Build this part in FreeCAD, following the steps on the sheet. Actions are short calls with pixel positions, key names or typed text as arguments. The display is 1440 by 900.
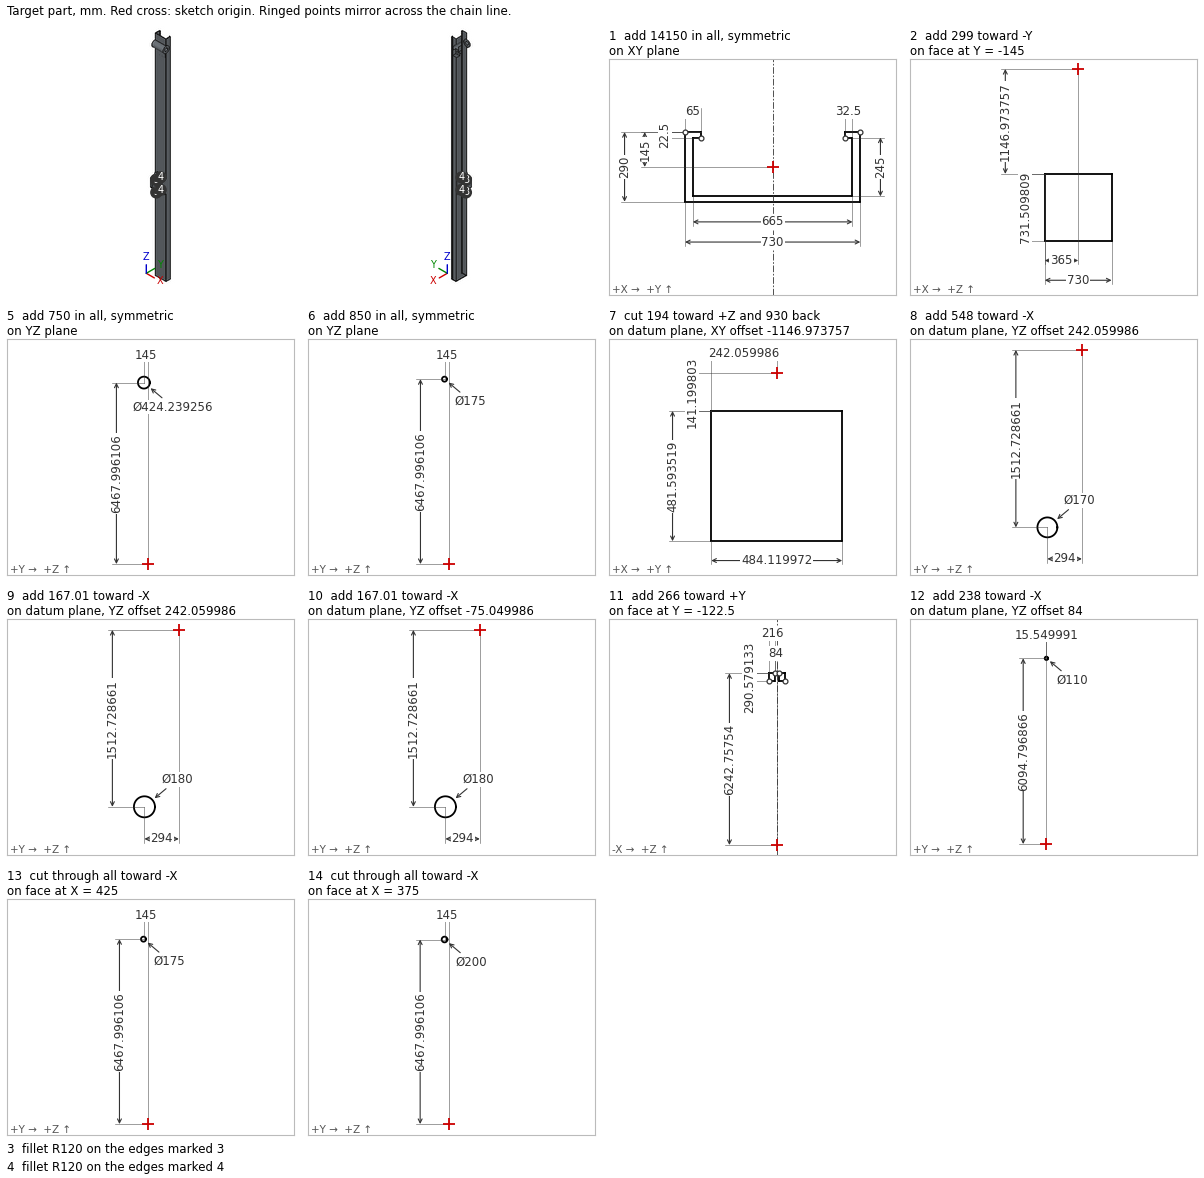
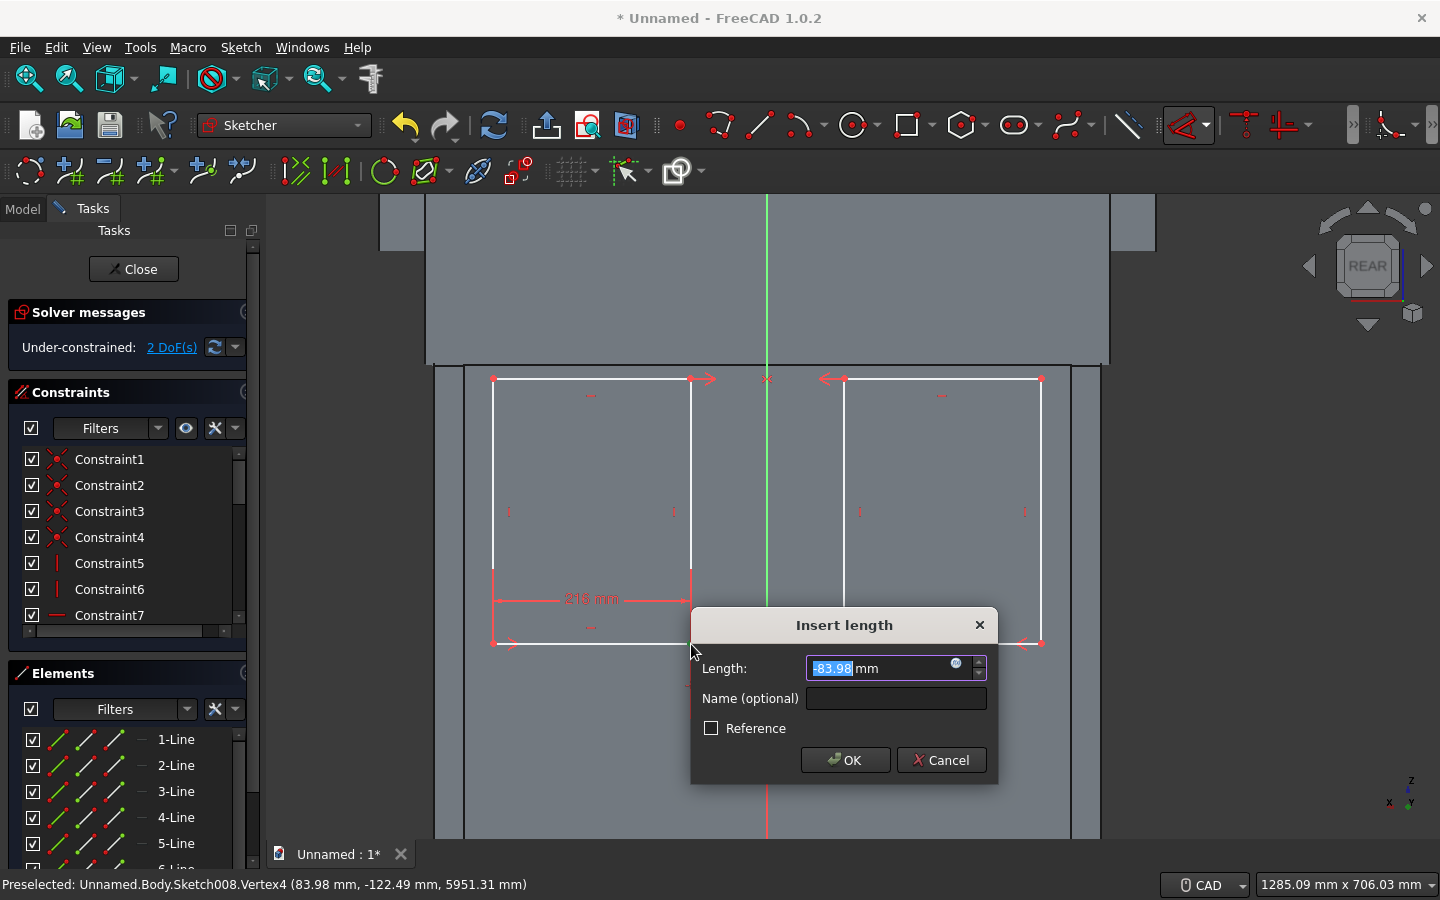
text(-84)
key(Return)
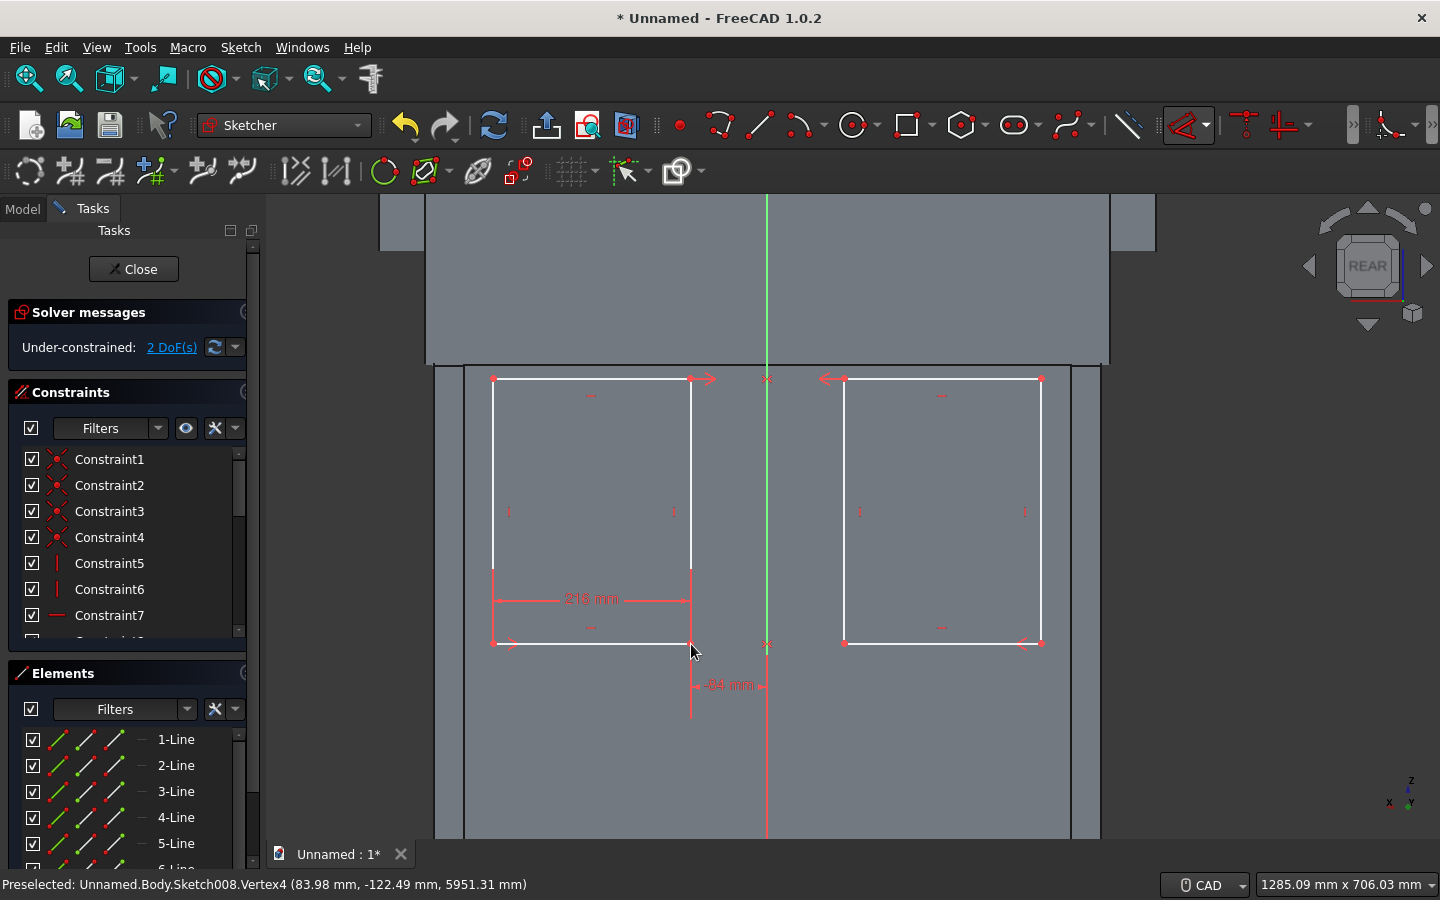
click(493, 459)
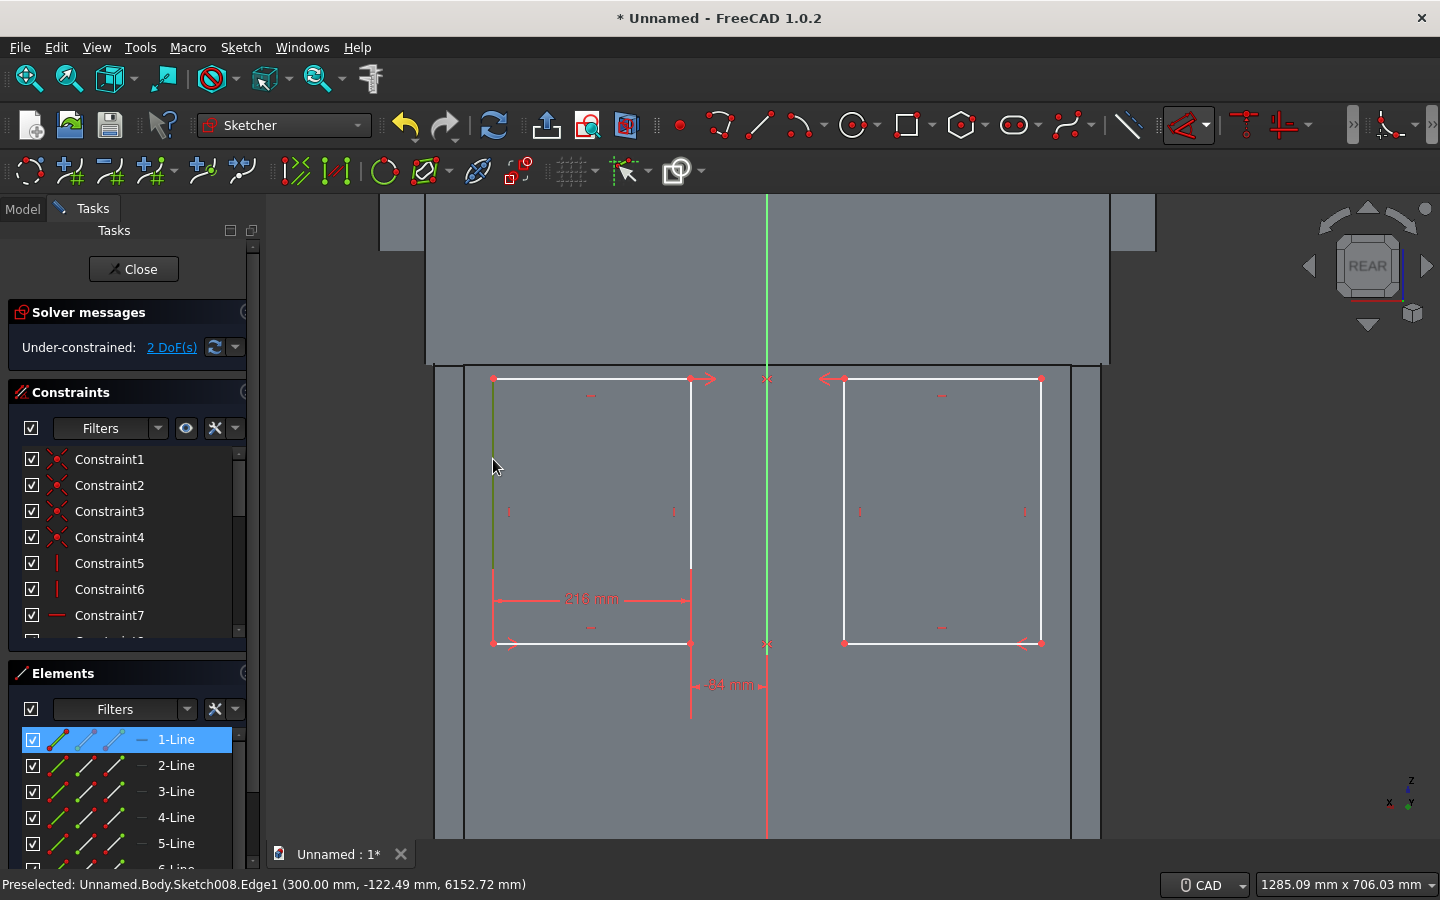
click(1208, 126)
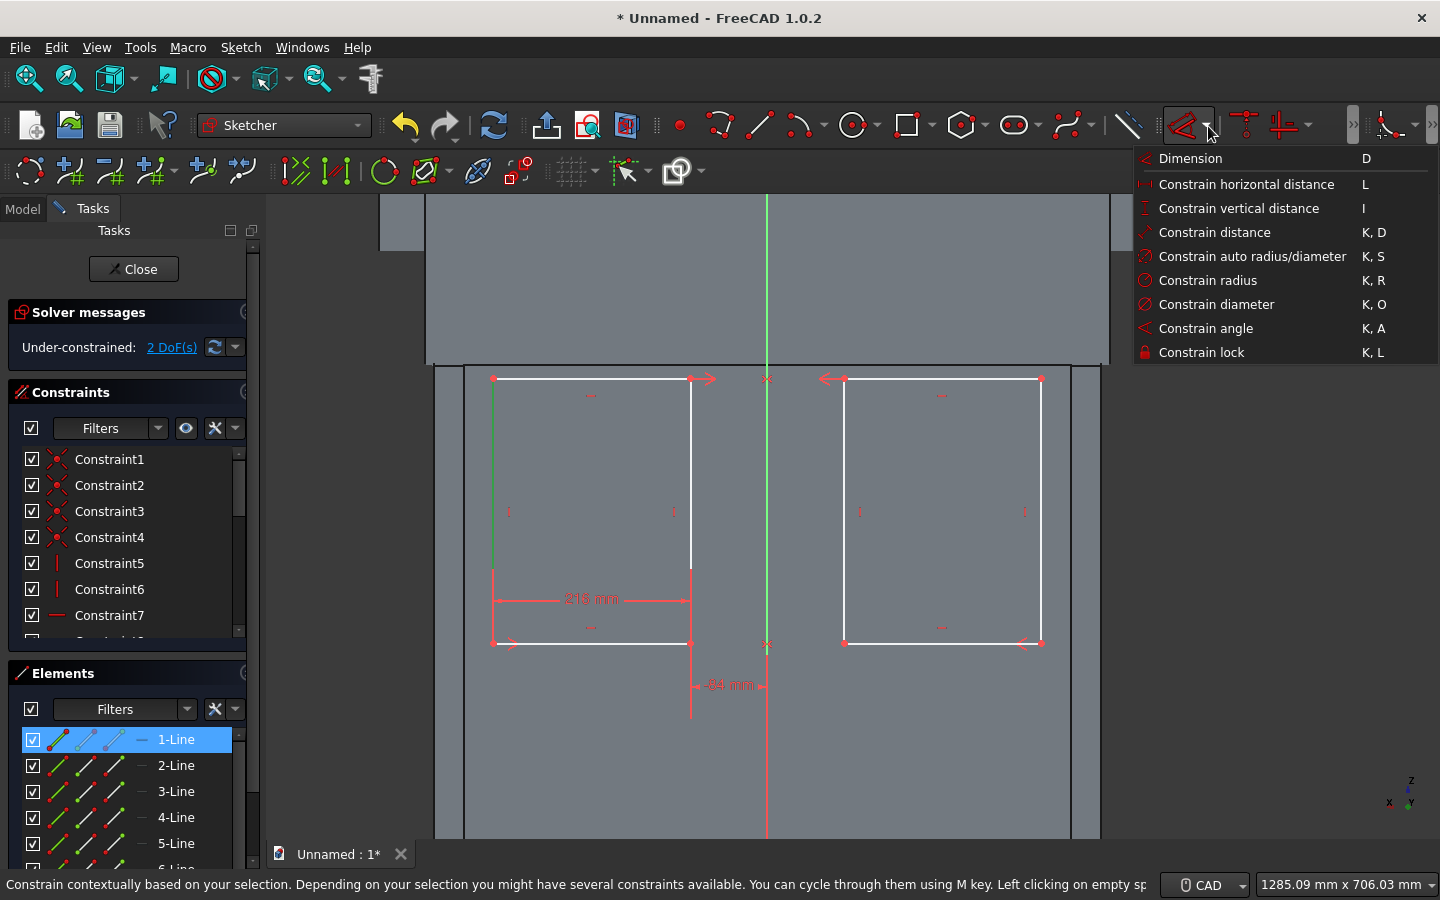
click(1286, 208)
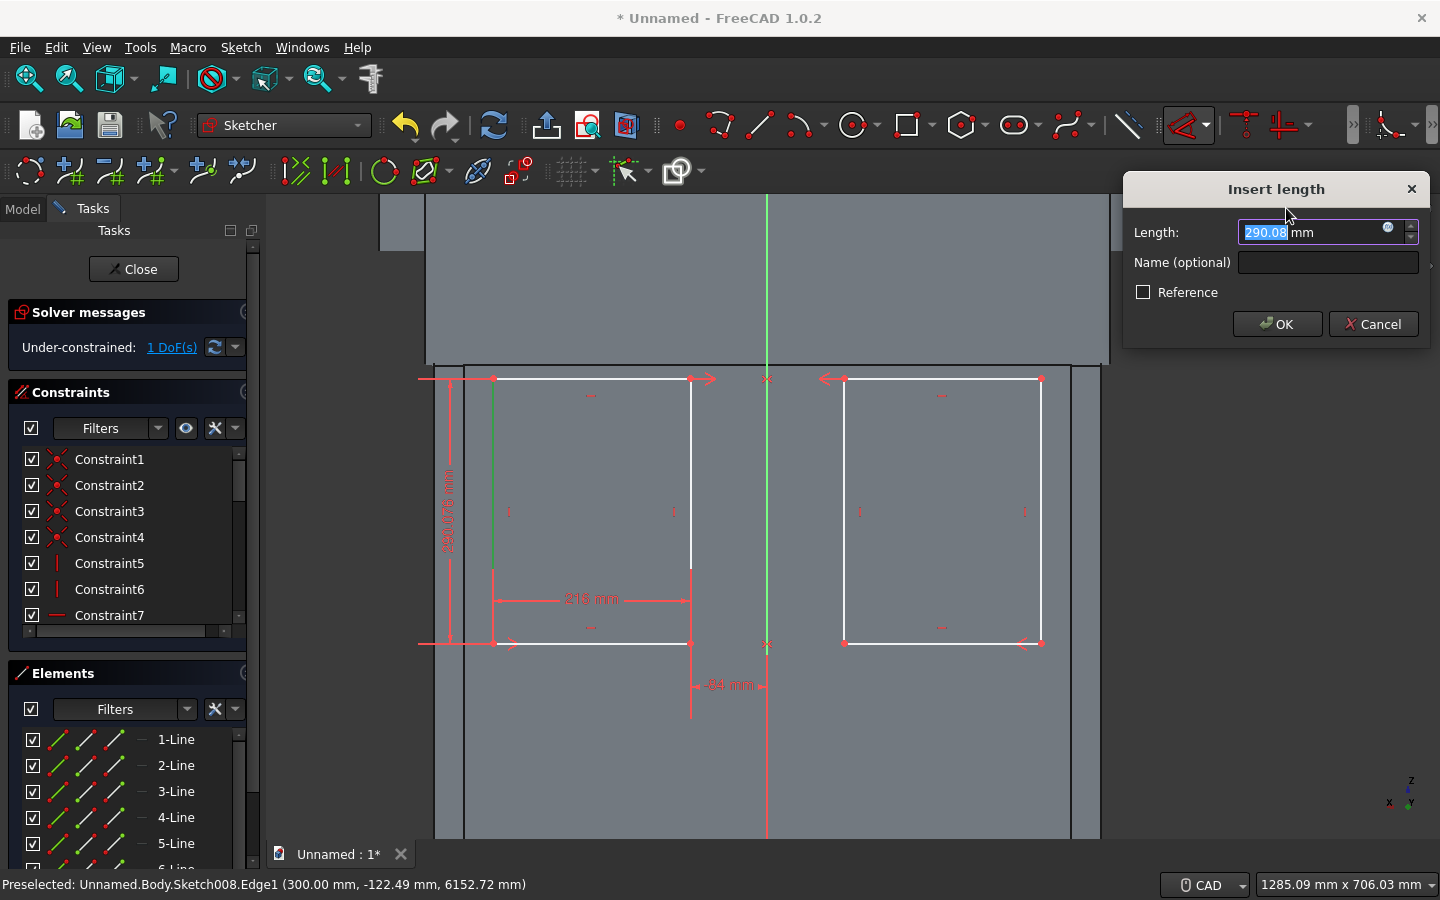
text(290.579133)
key(Return)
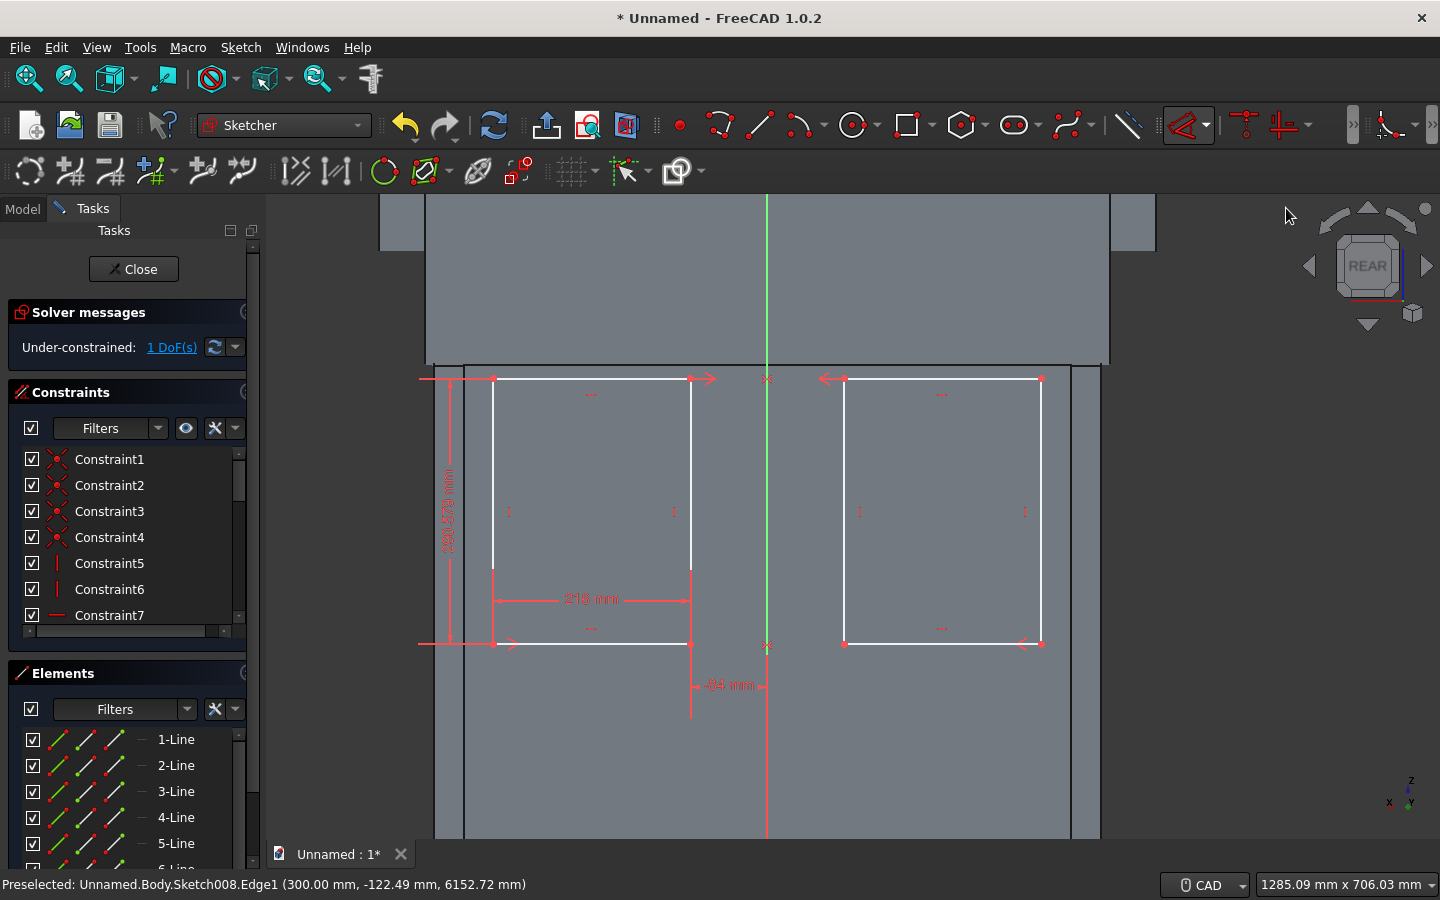
click(493, 379)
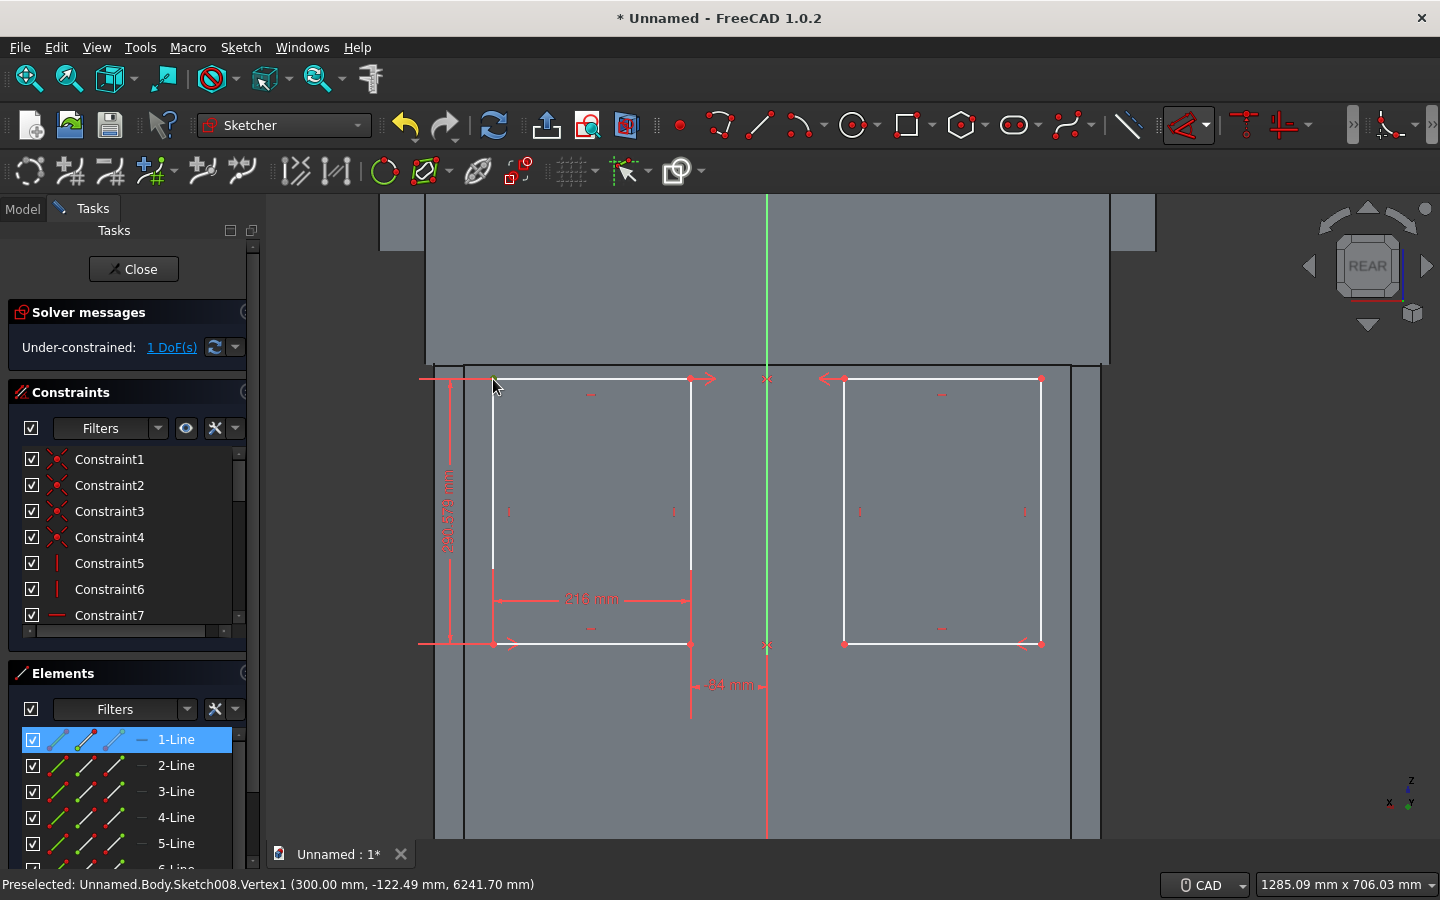
key(i)